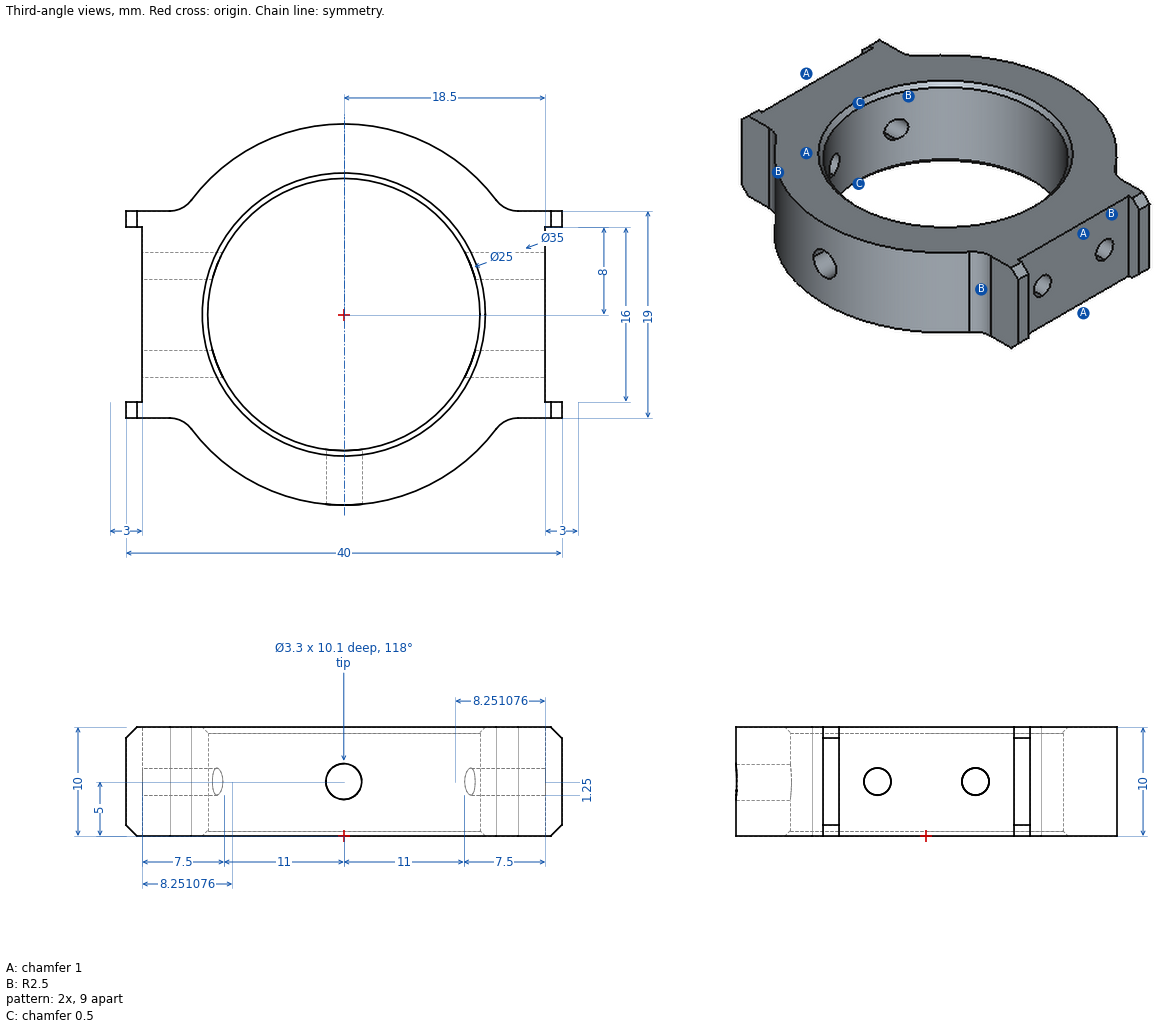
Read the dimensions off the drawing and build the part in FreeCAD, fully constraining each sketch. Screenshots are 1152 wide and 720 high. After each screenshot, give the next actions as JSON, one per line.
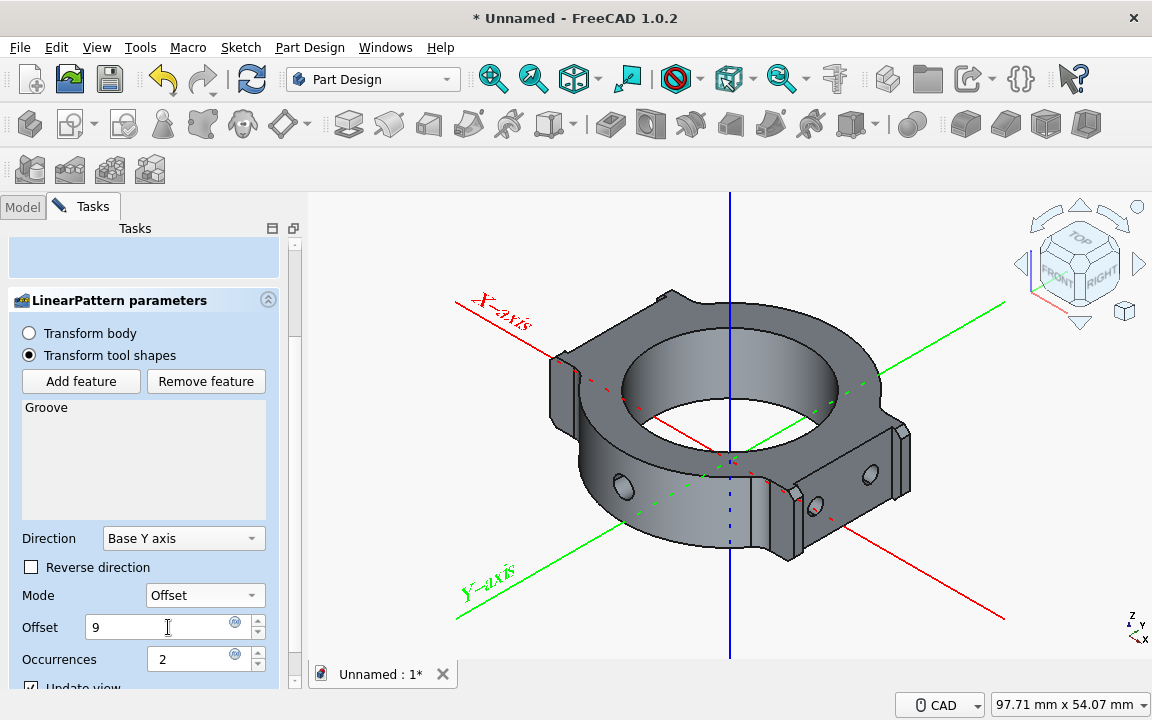
{"action": "triple_click", "coordinate": [198, 659]}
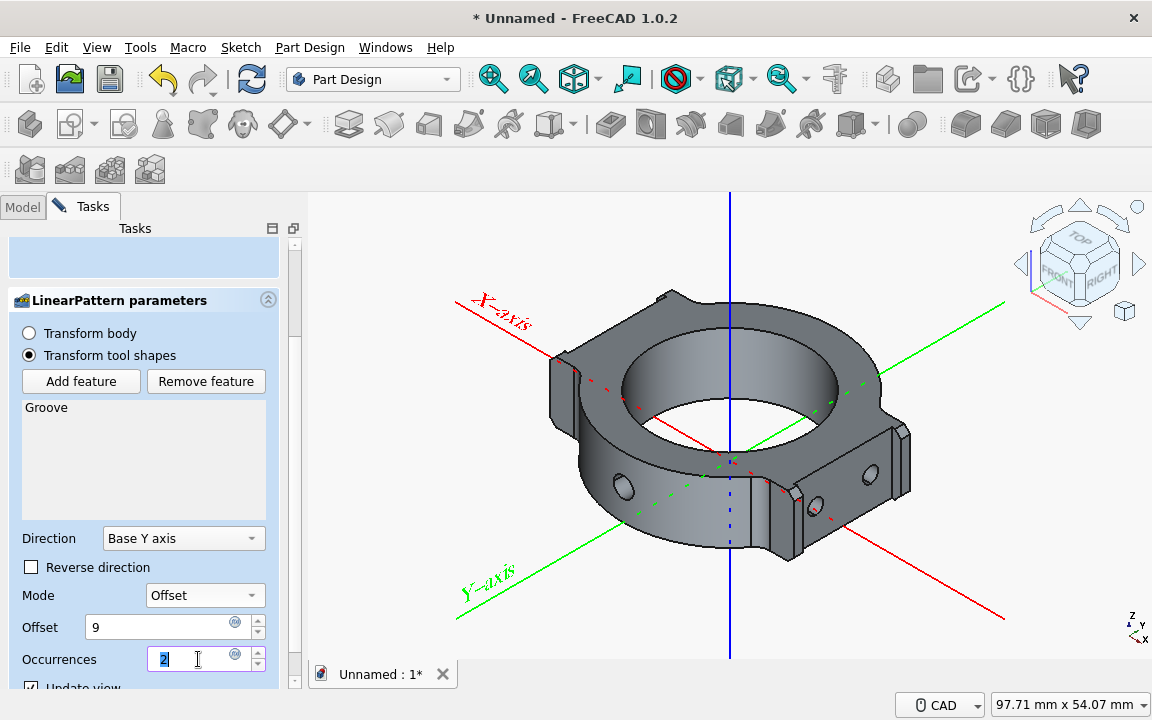
{"action": "type", "text": "2"}
{"action": "key", "text": "Tab"}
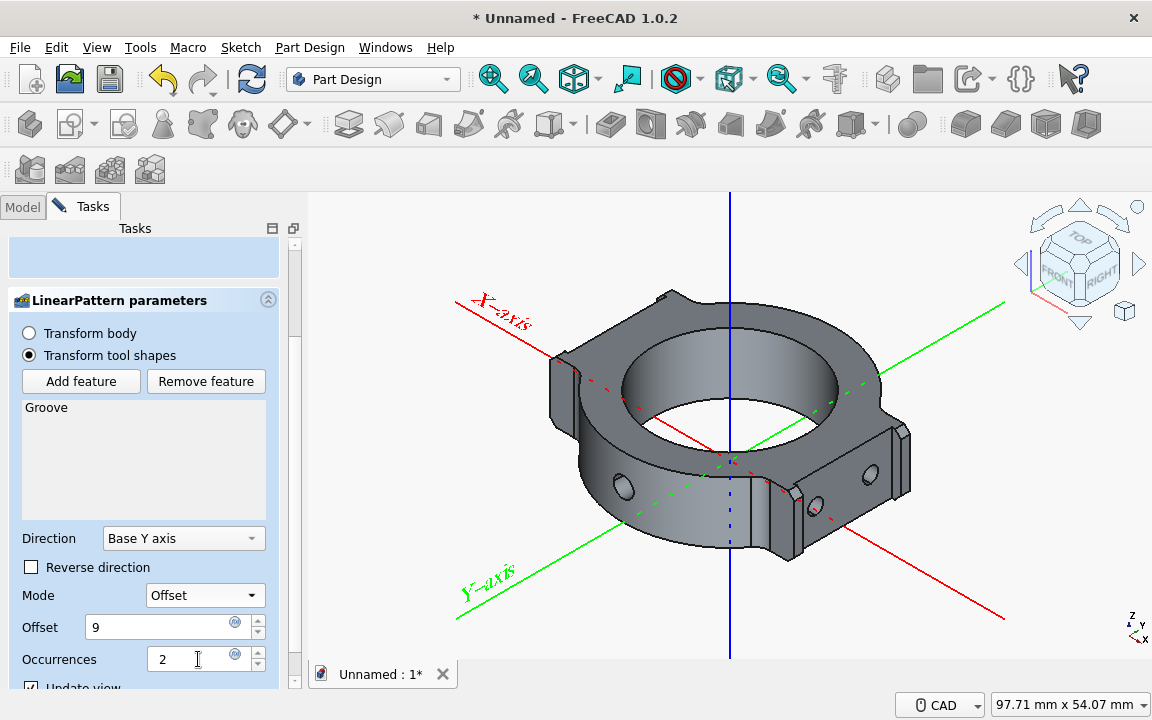
{"action": "scroll", "coordinate": [295, 463], "scroll_direction": "up", "scroll_amount": 3}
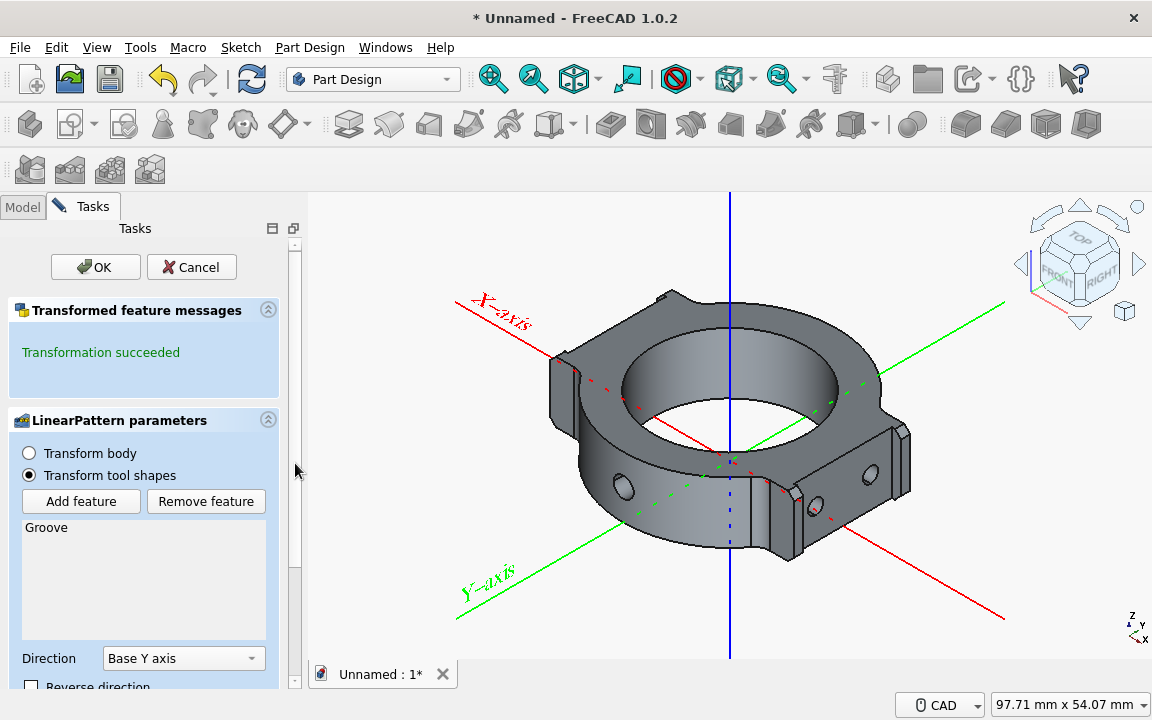
{"action": "left_click", "coordinate": [96, 267]}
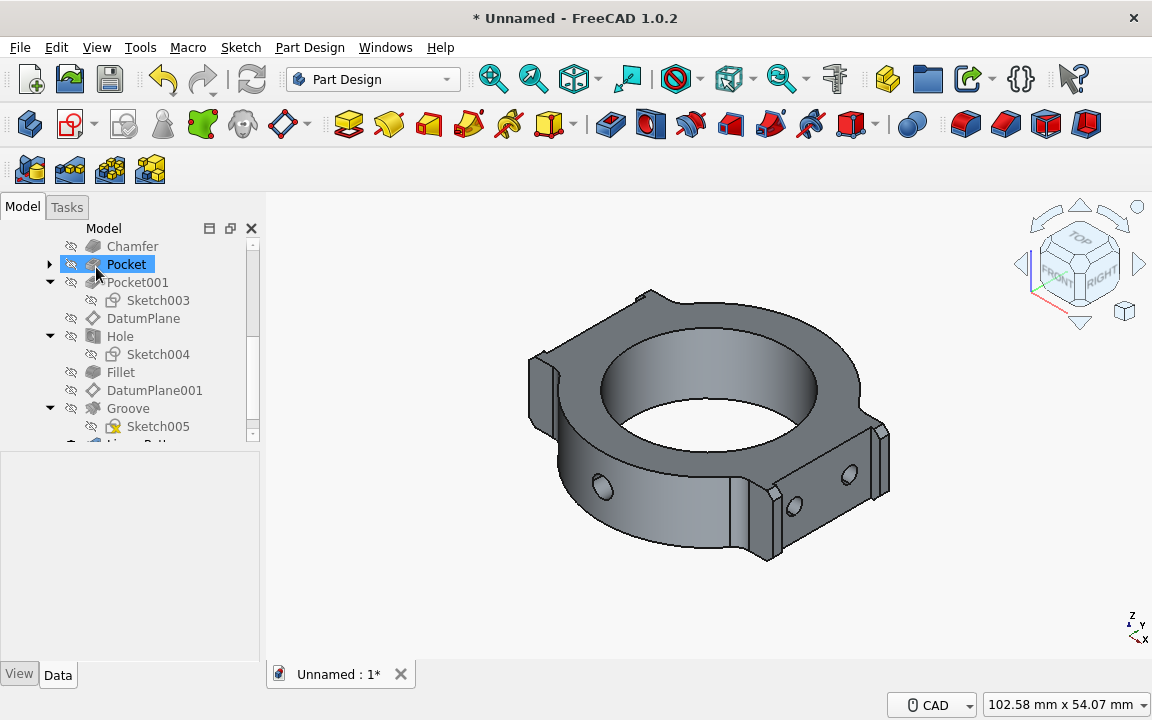
{"action": "left_click", "coordinate": [116, 408]}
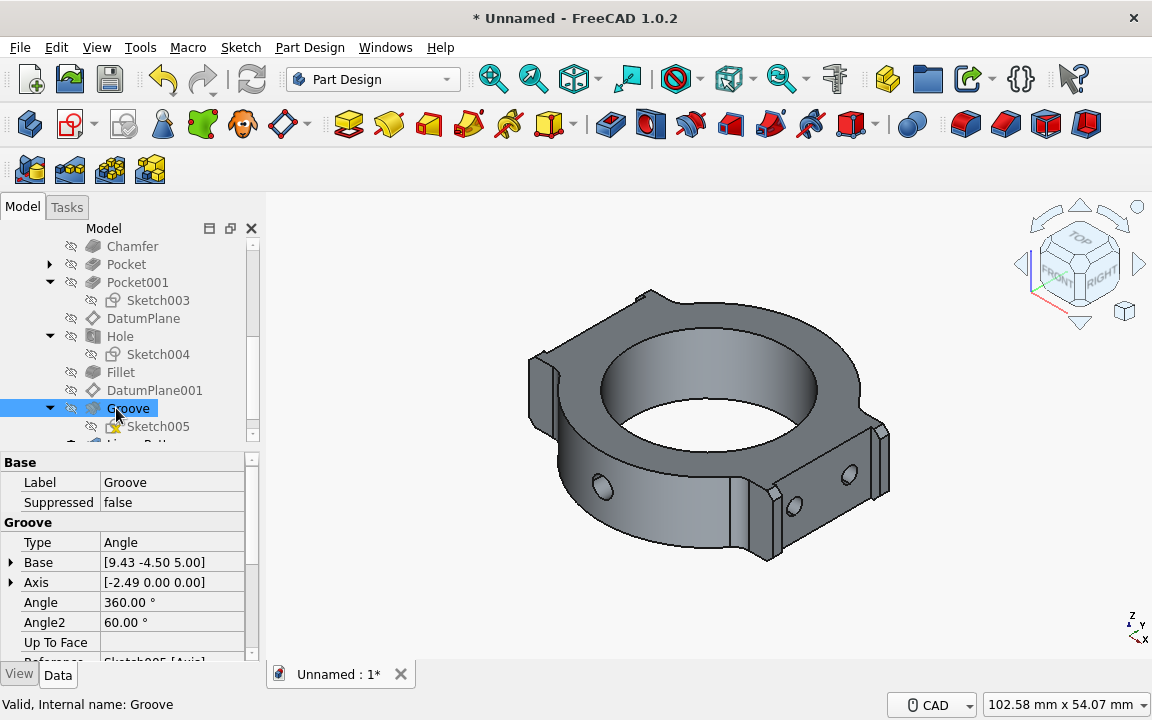
{"action": "left_click", "coordinate": [30, 170]}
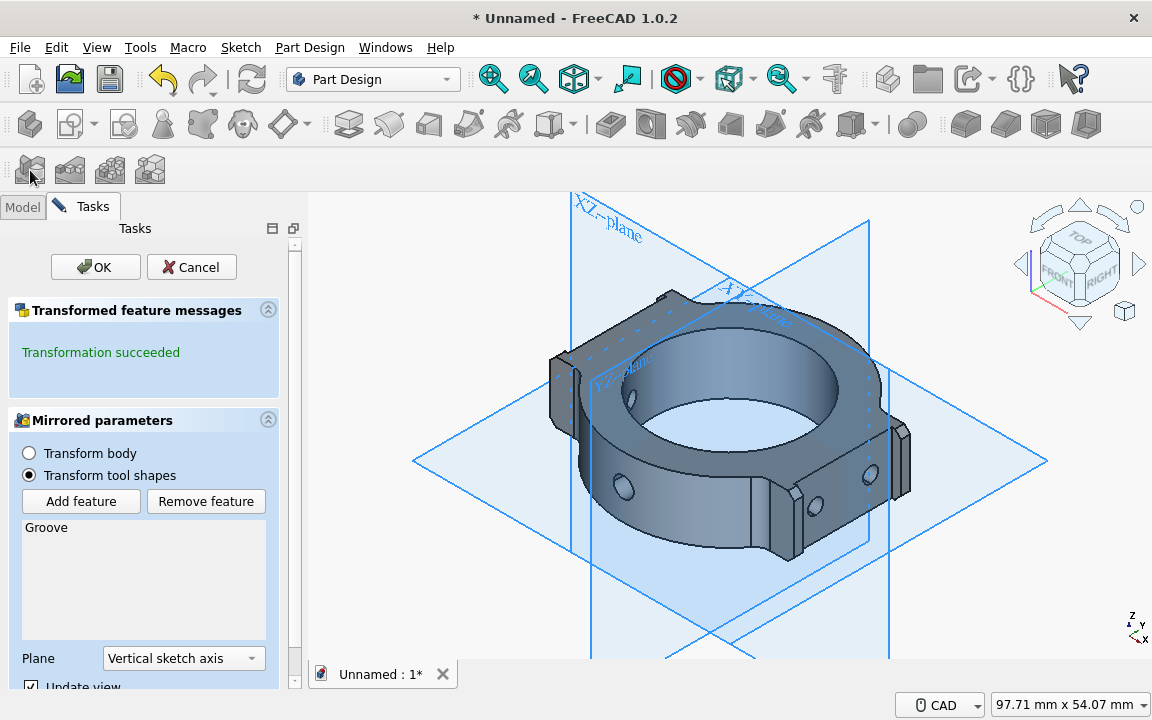
{"action": "left_click", "coordinate": [184, 658]}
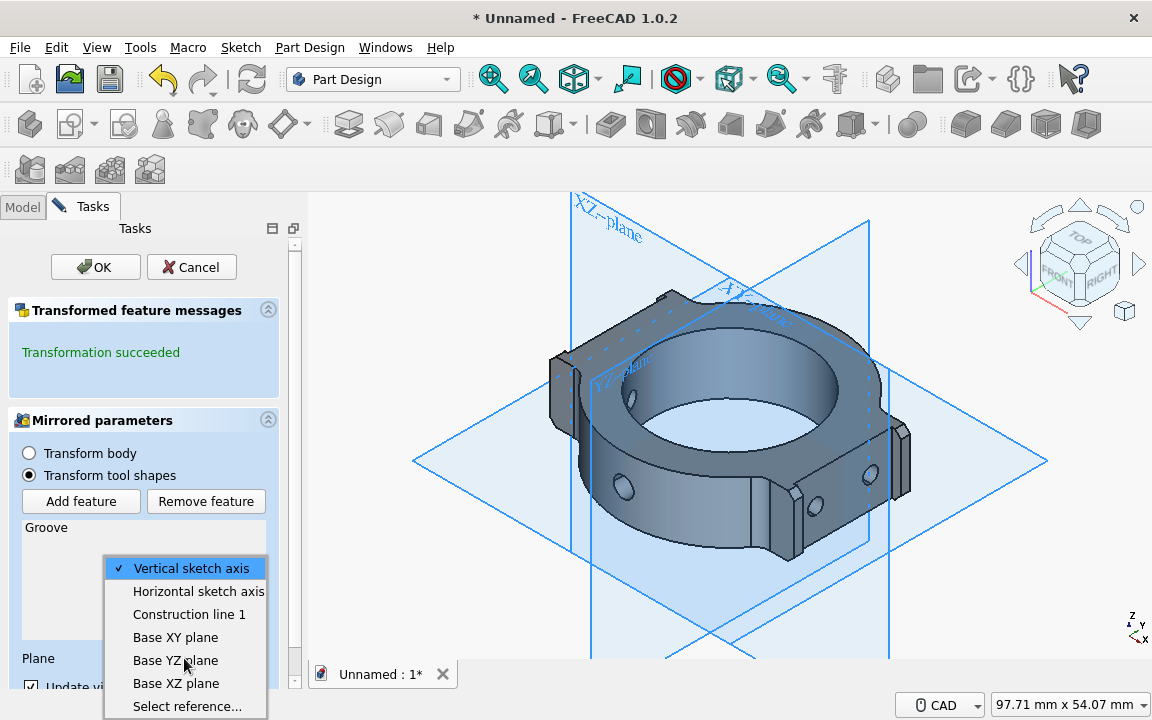
{"action": "left_click", "coordinate": [184, 660]}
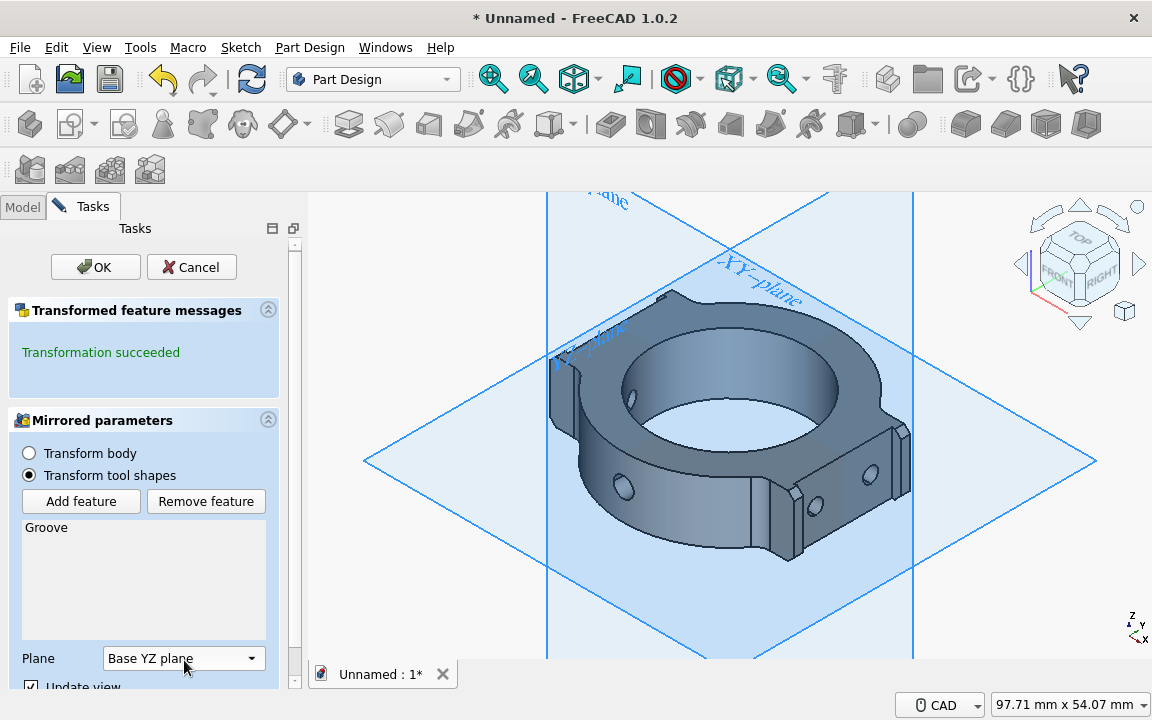
{"action": "left_click", "coordinate": [96, 267]}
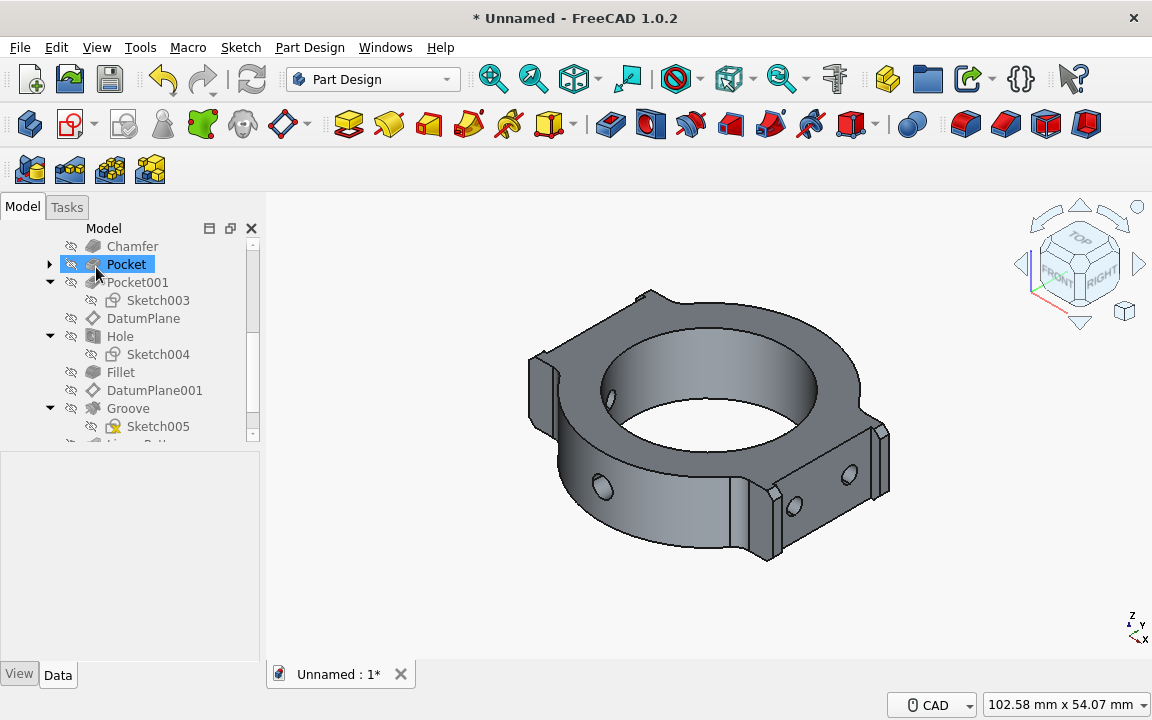
{"action": "scroll", "coordinate": [140, 332], "scroll_direction": "down", "scroll_amount": 3}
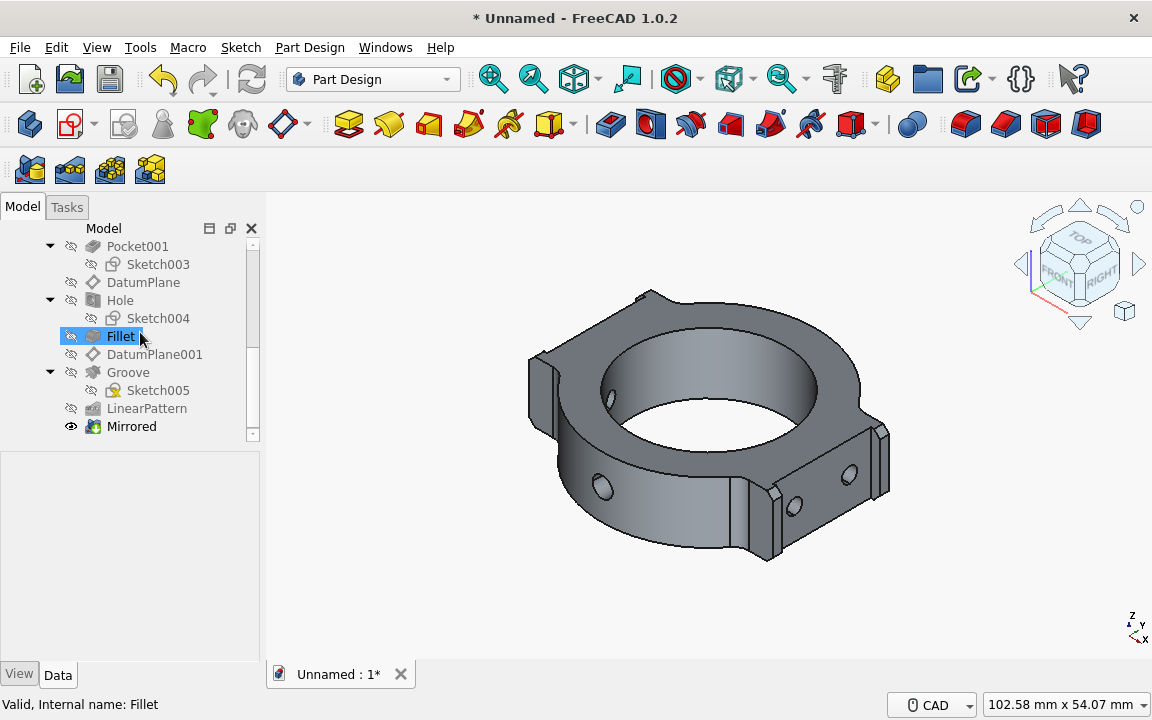
{"action": "scroll", "coordinate": [140, 332], "scroll_direction": "up", "scroll_amount": 15}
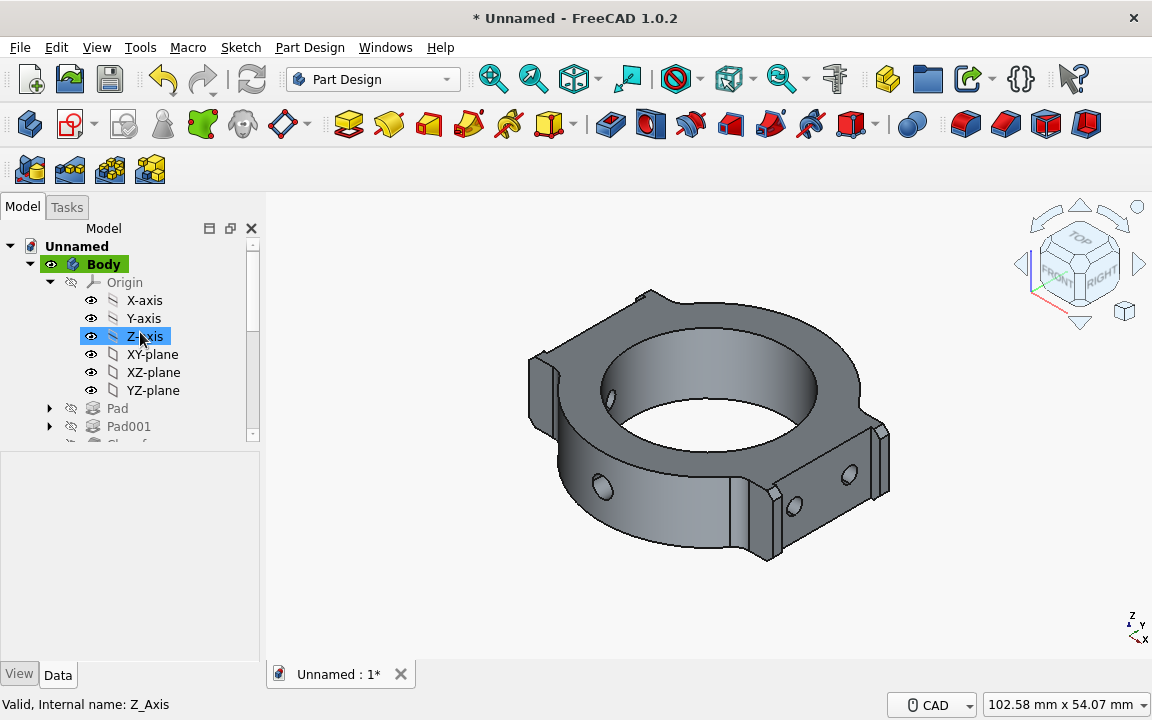
{"action": "left_click", "coordinate": [136, 372]}